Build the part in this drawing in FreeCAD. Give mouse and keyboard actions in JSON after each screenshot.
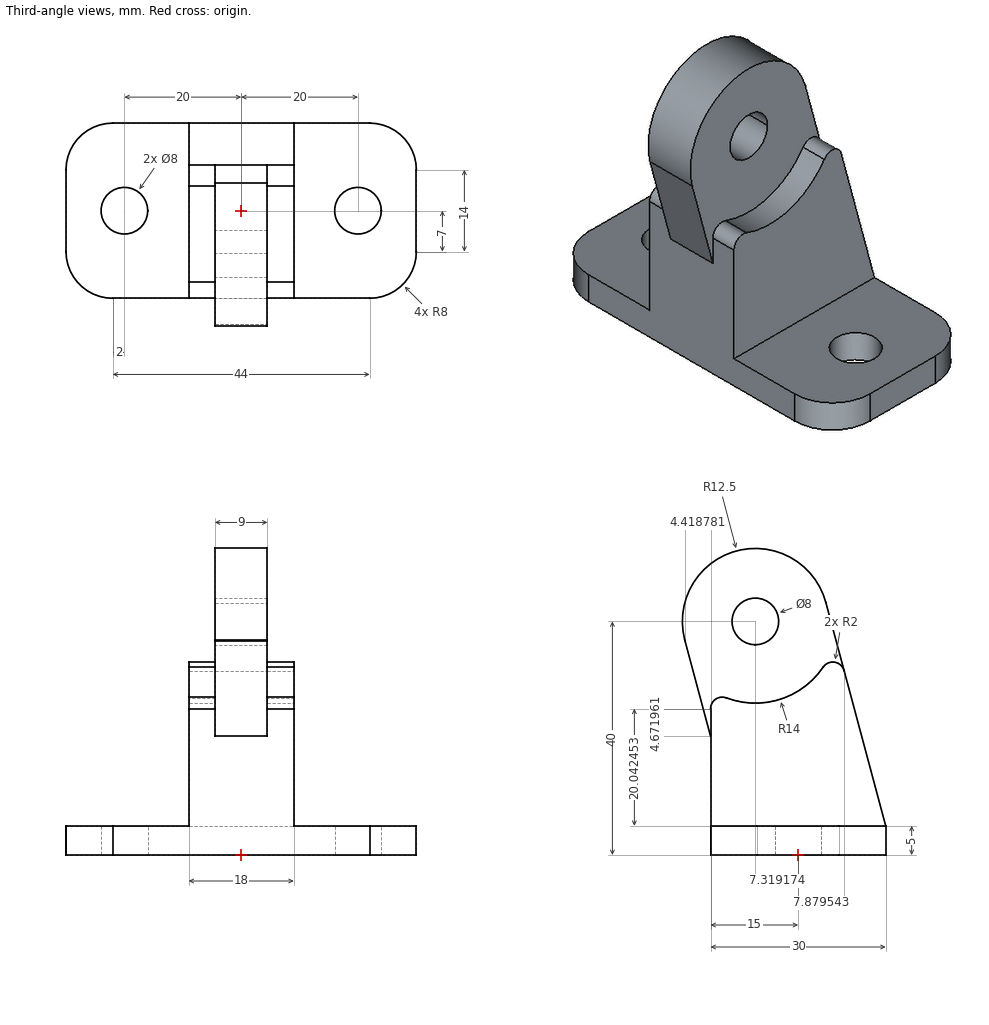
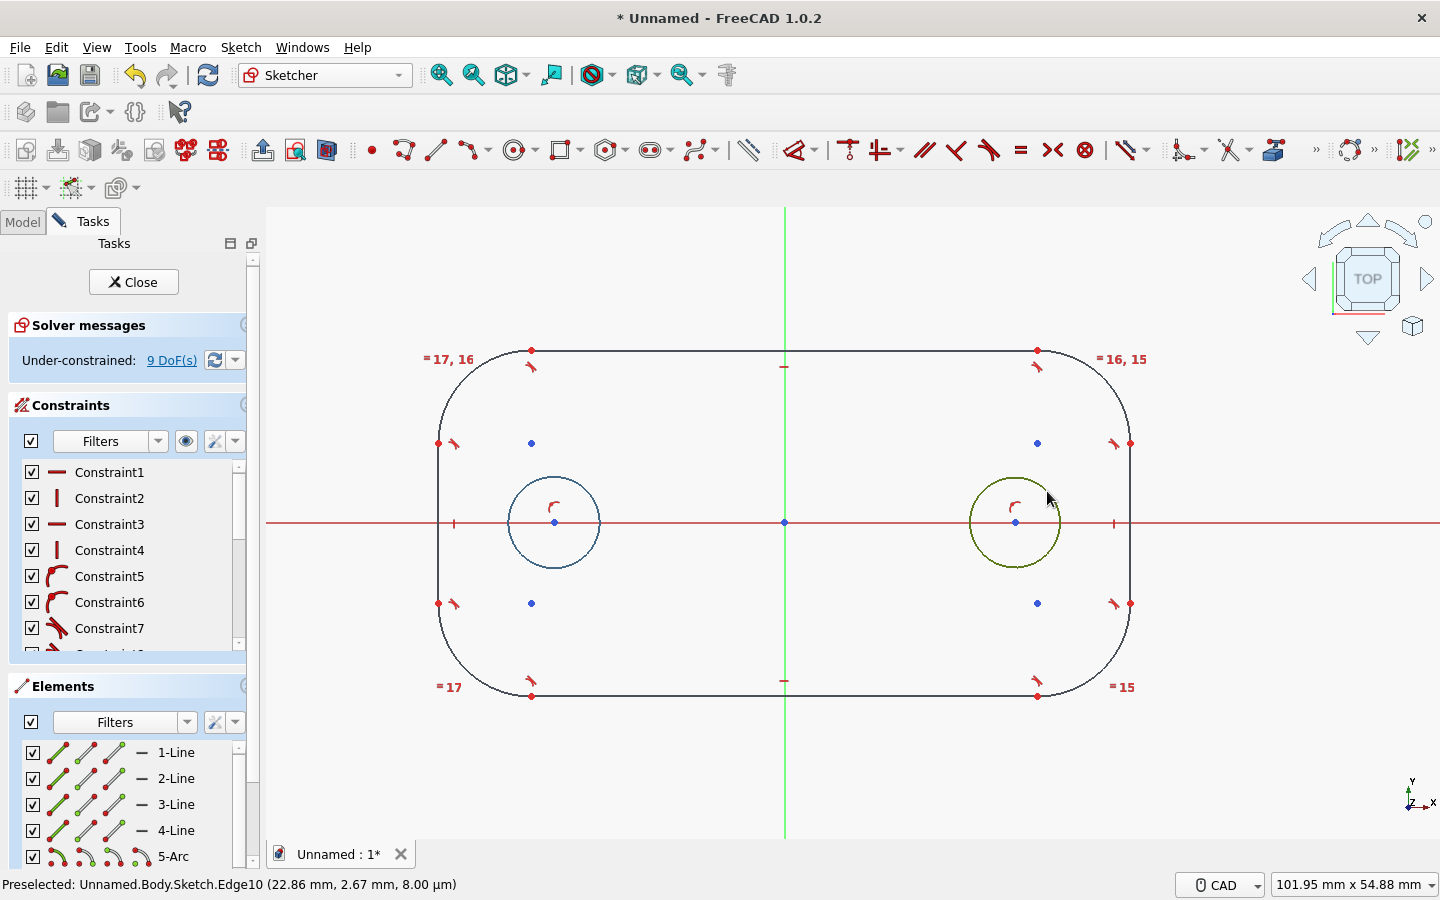
{"action": "key", "text": "e"}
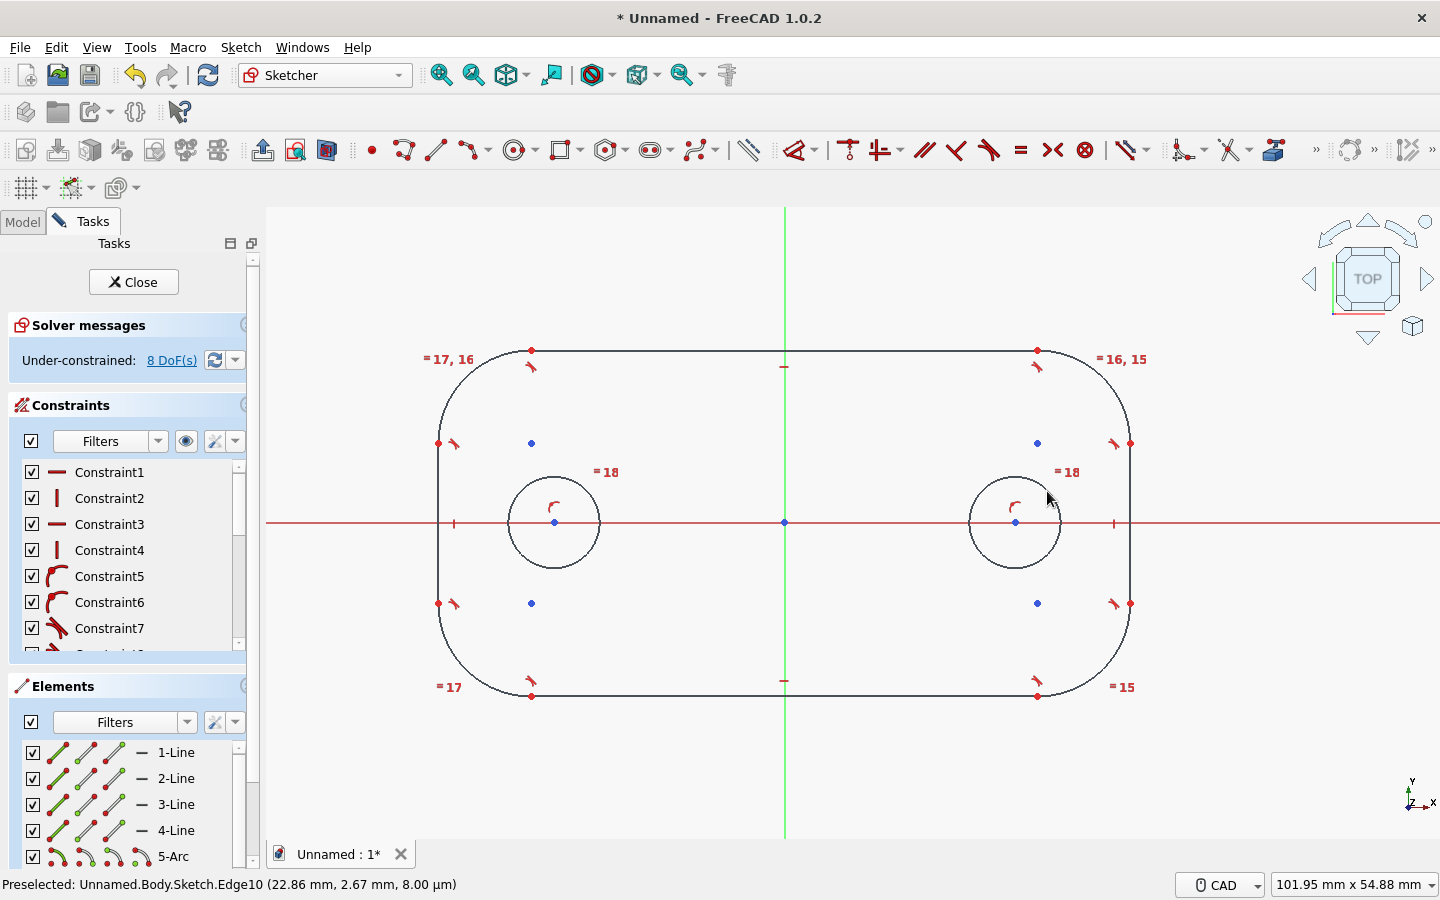
{"action": "left_click", "coordinate": [1080, 686]}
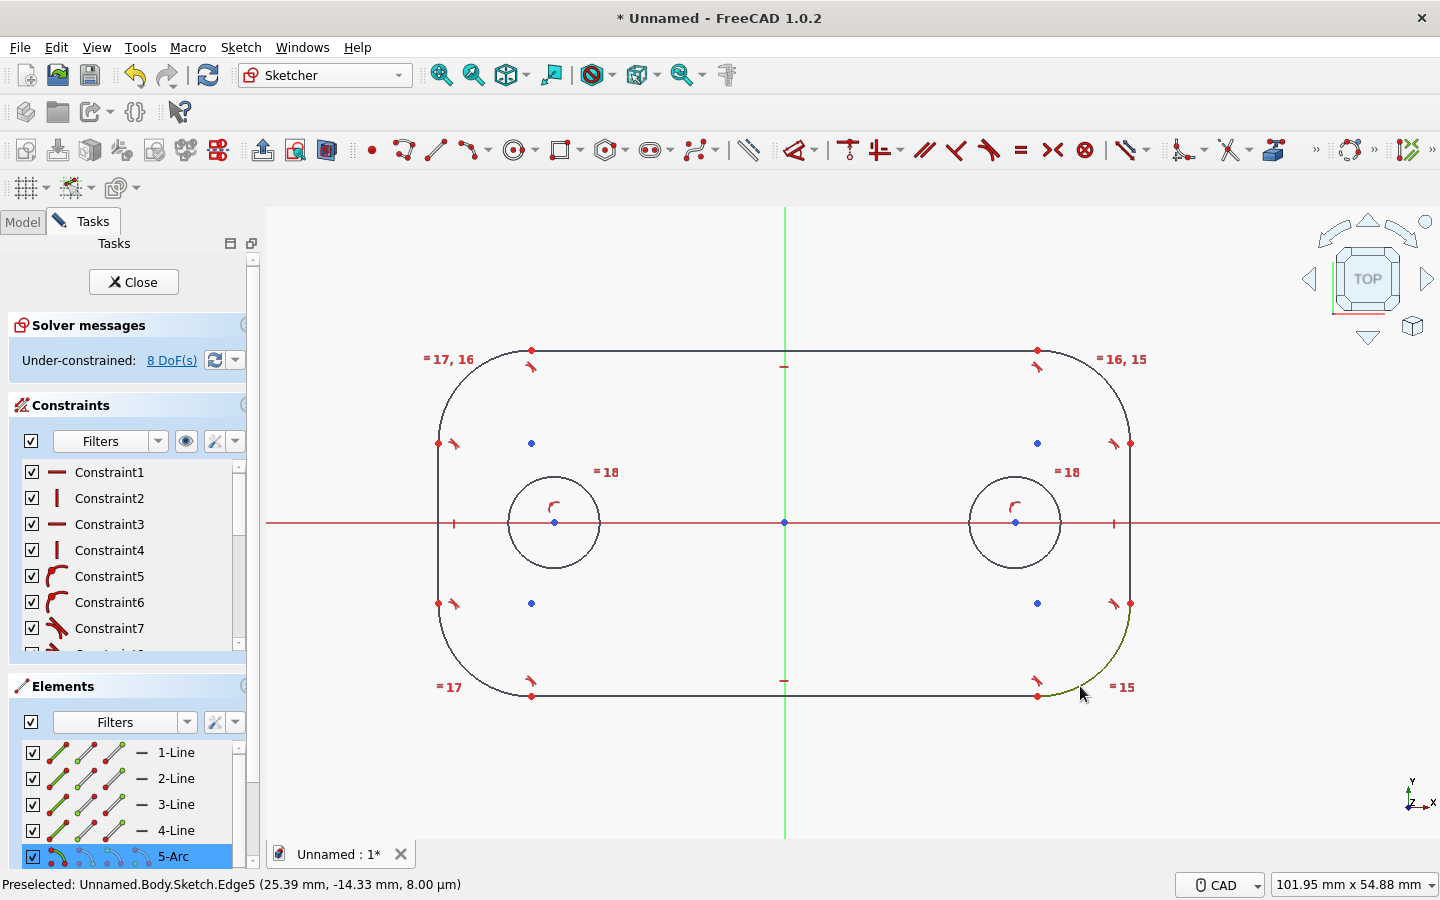
{"action": "left_click", "coordinate": [816, 150]}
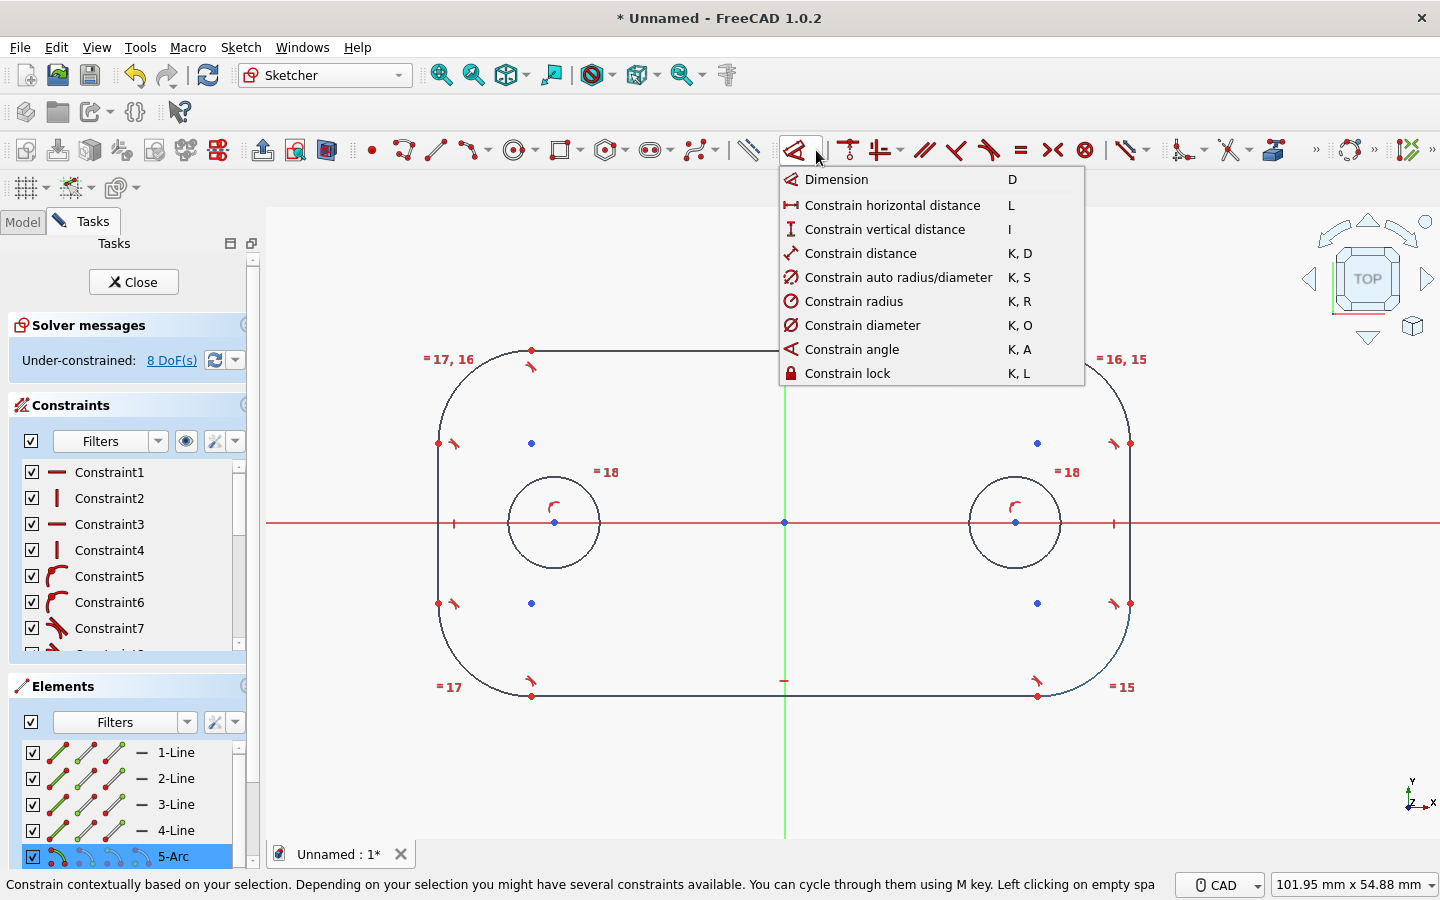
{"action": "left_click", "coordinate": [932, 301]}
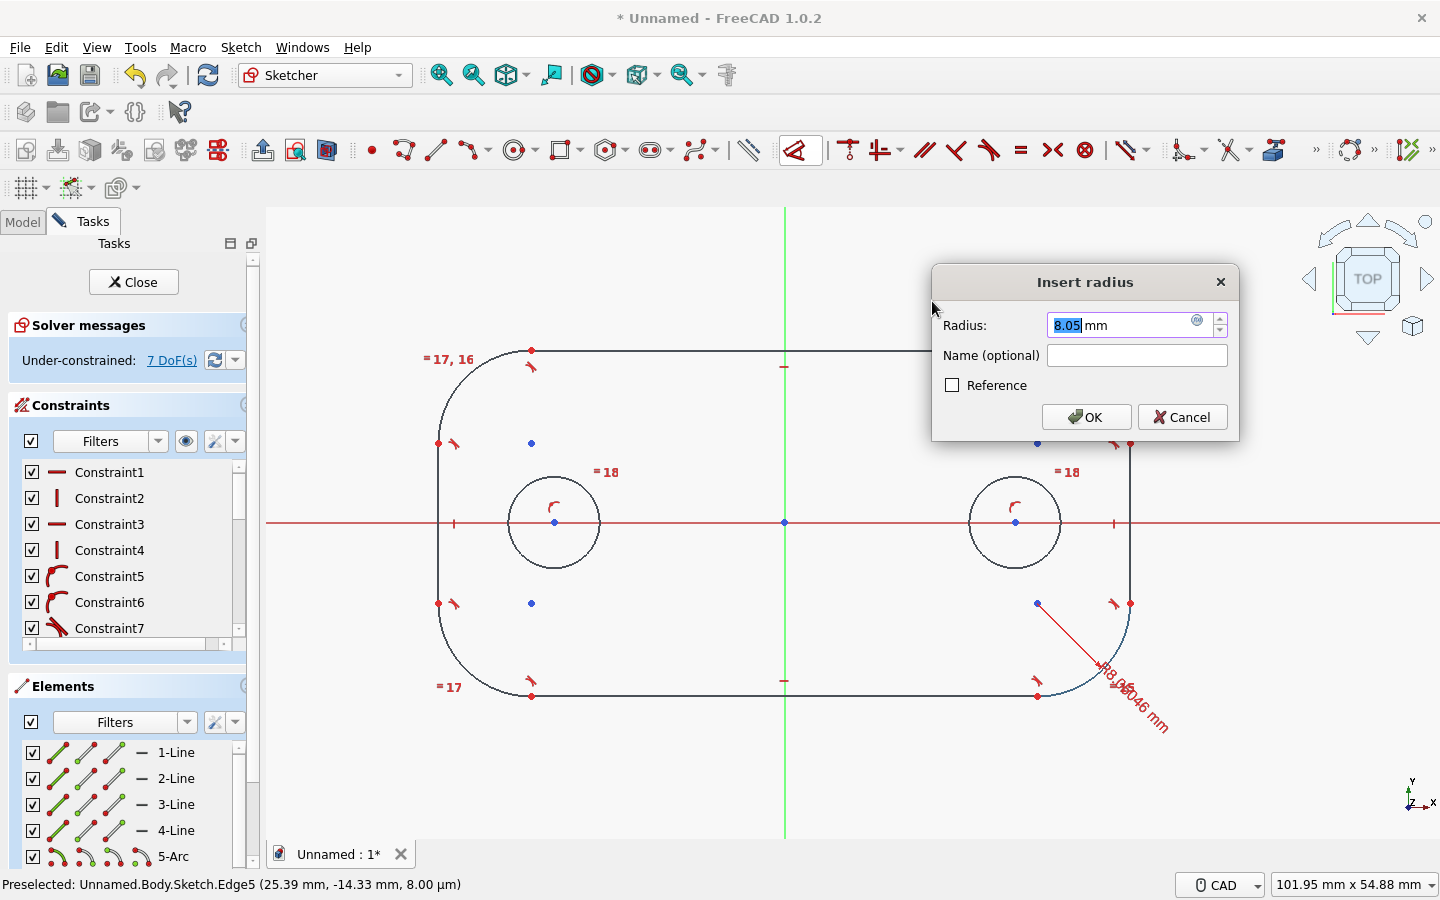
{"action": "type", "text": "8"}
{"action": "key", "text": "Return"}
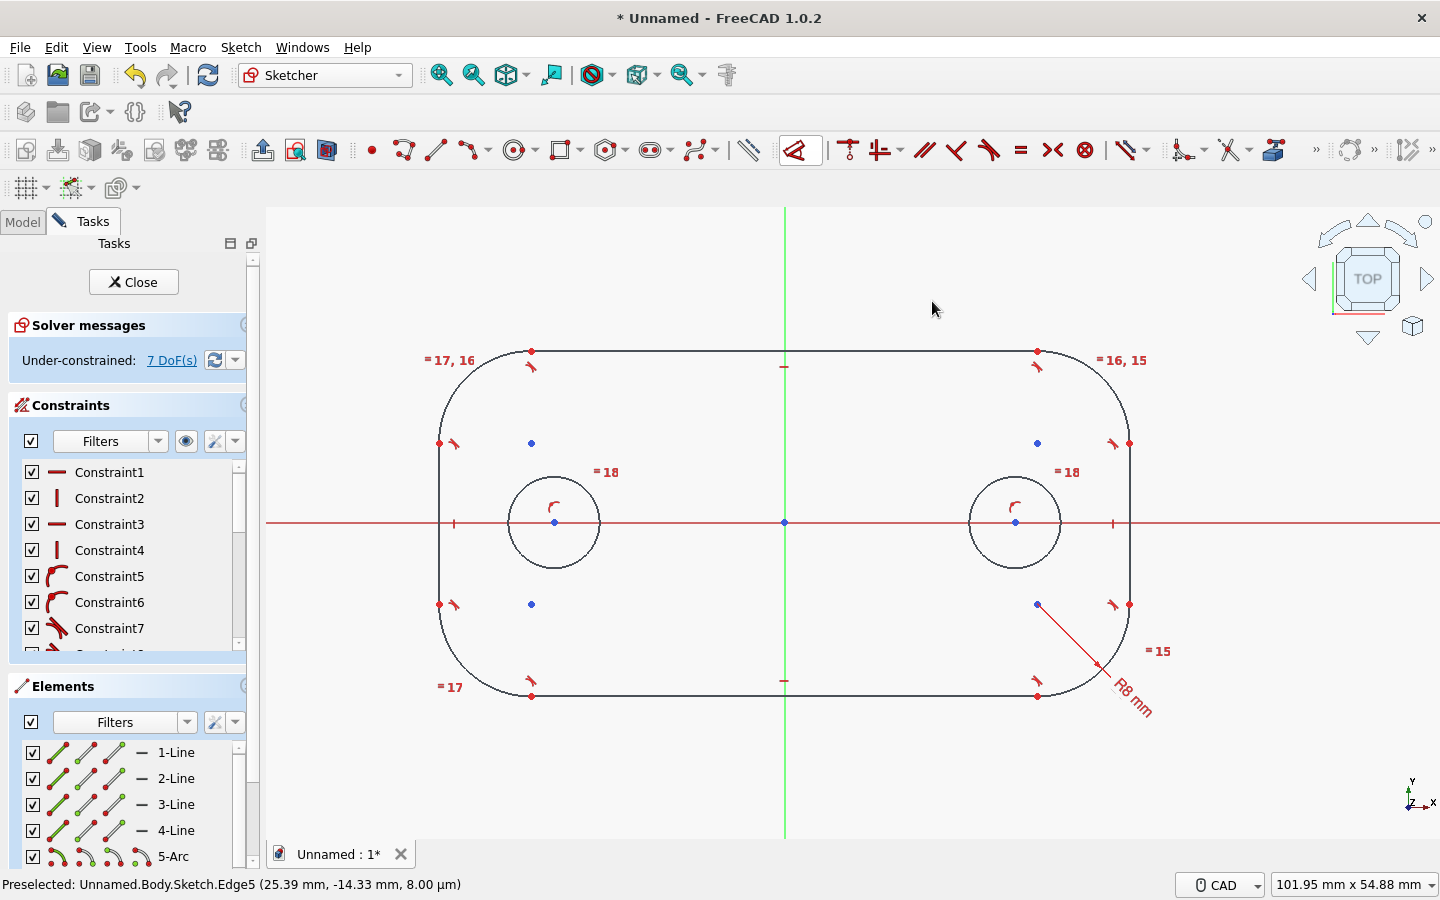
{"action": "left_click", "coordinate": [586, 490]}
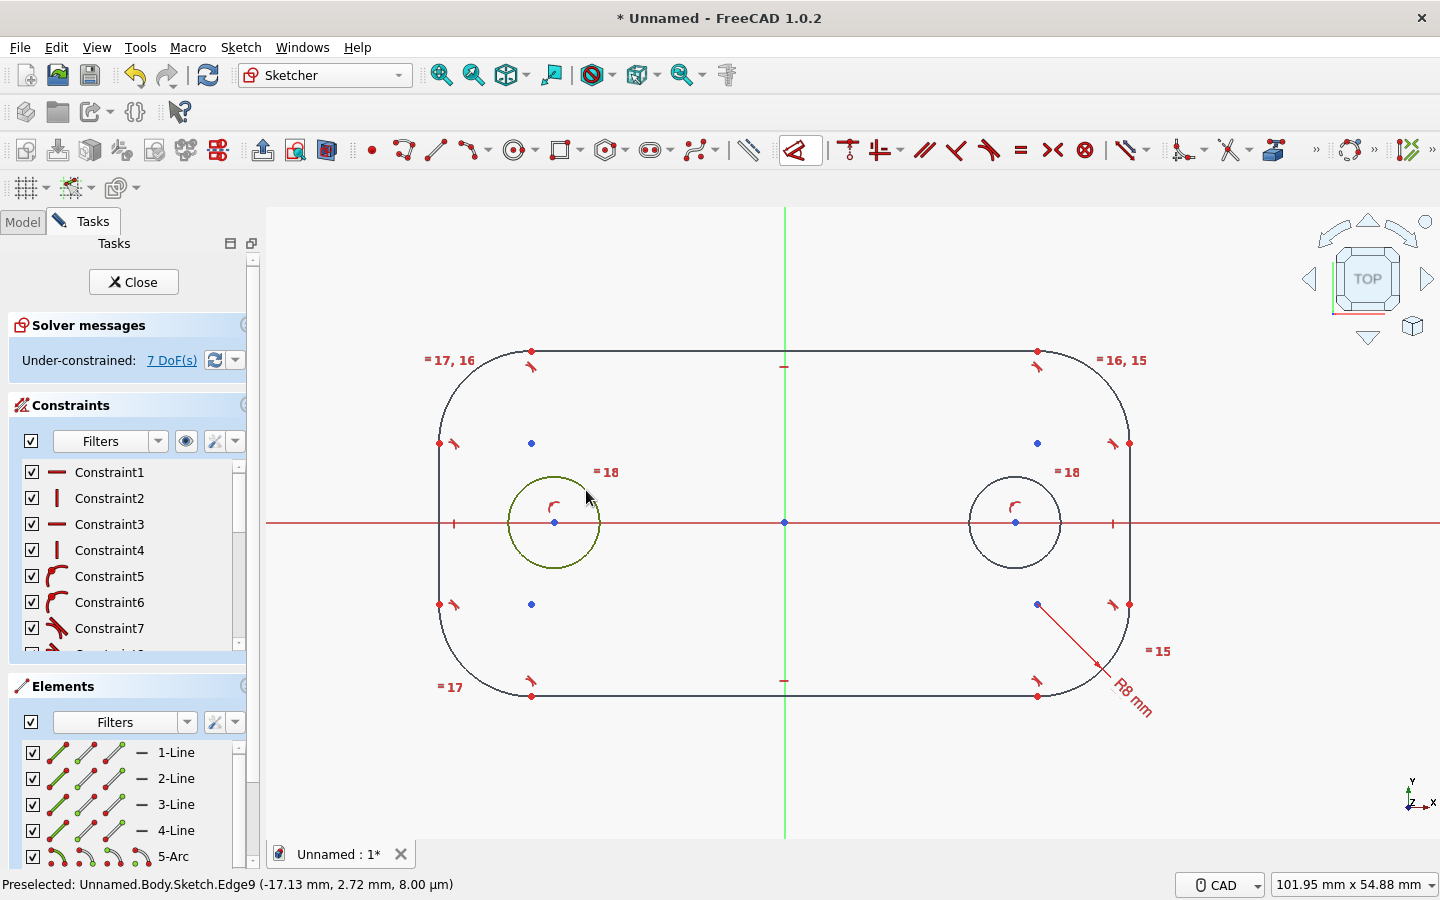
{"action": "key", "text": "k o"}